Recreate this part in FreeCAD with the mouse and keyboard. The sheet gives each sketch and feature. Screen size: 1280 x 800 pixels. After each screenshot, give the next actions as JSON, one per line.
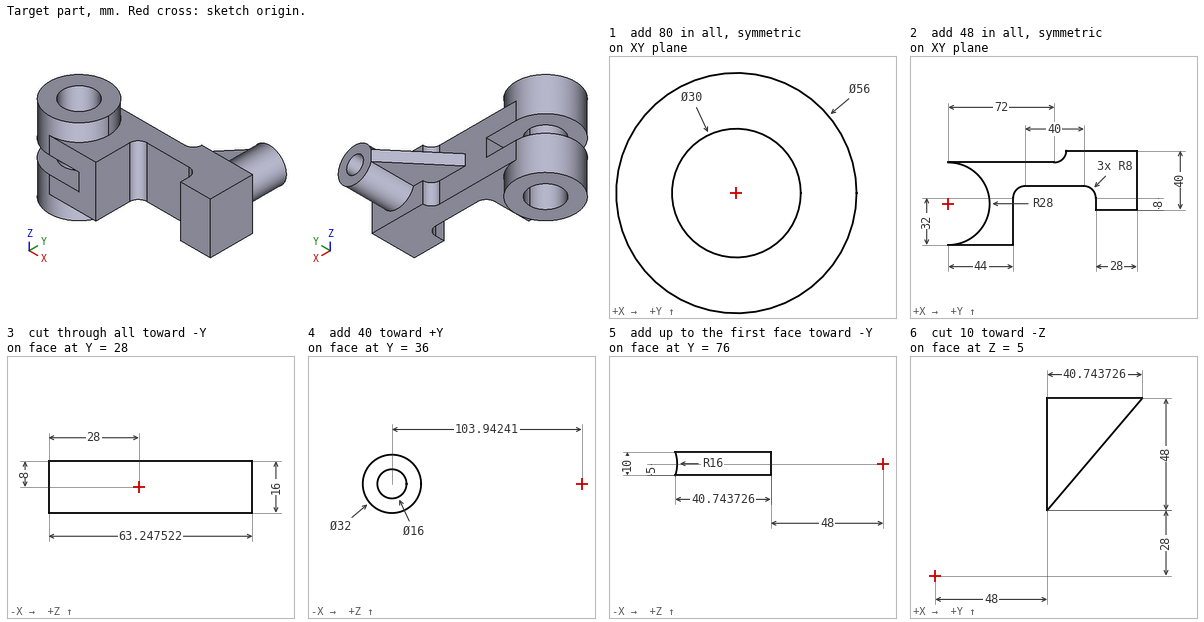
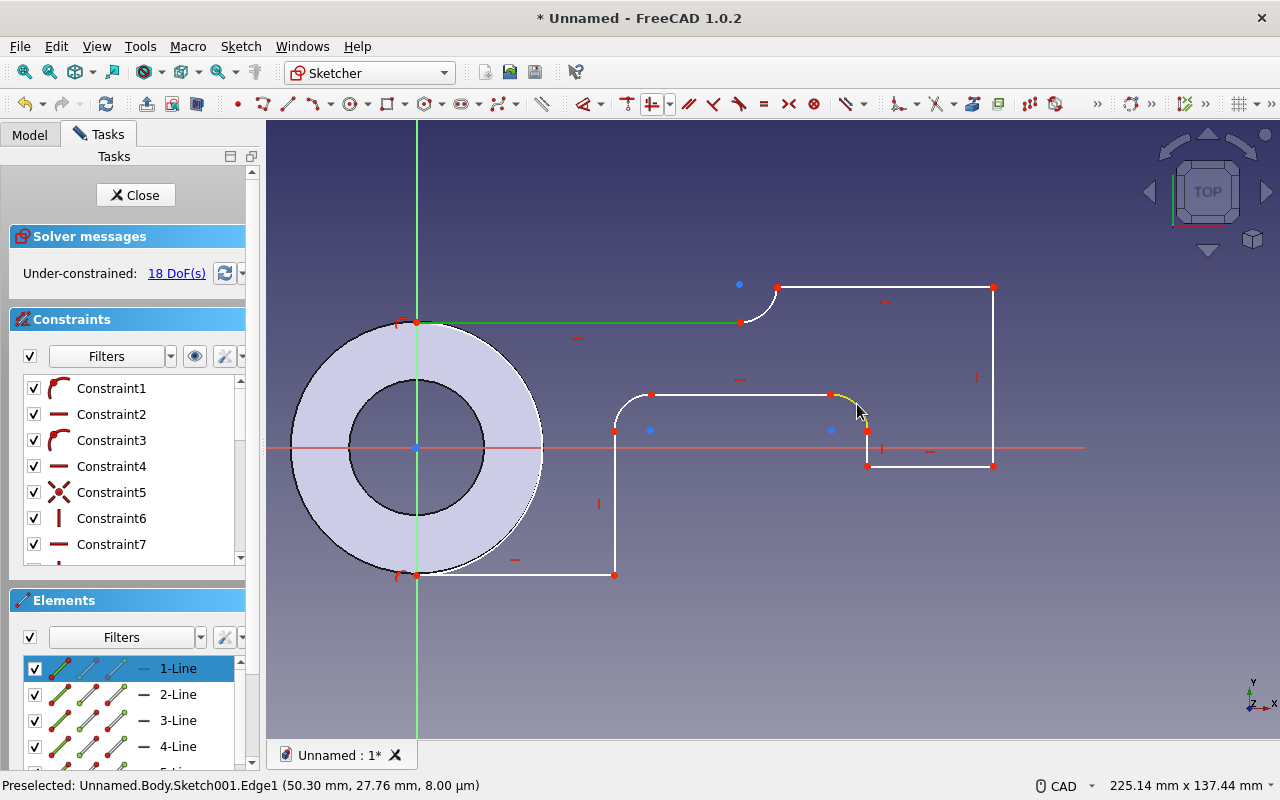
{"action": "left_click", "coordinate": [518, 523]}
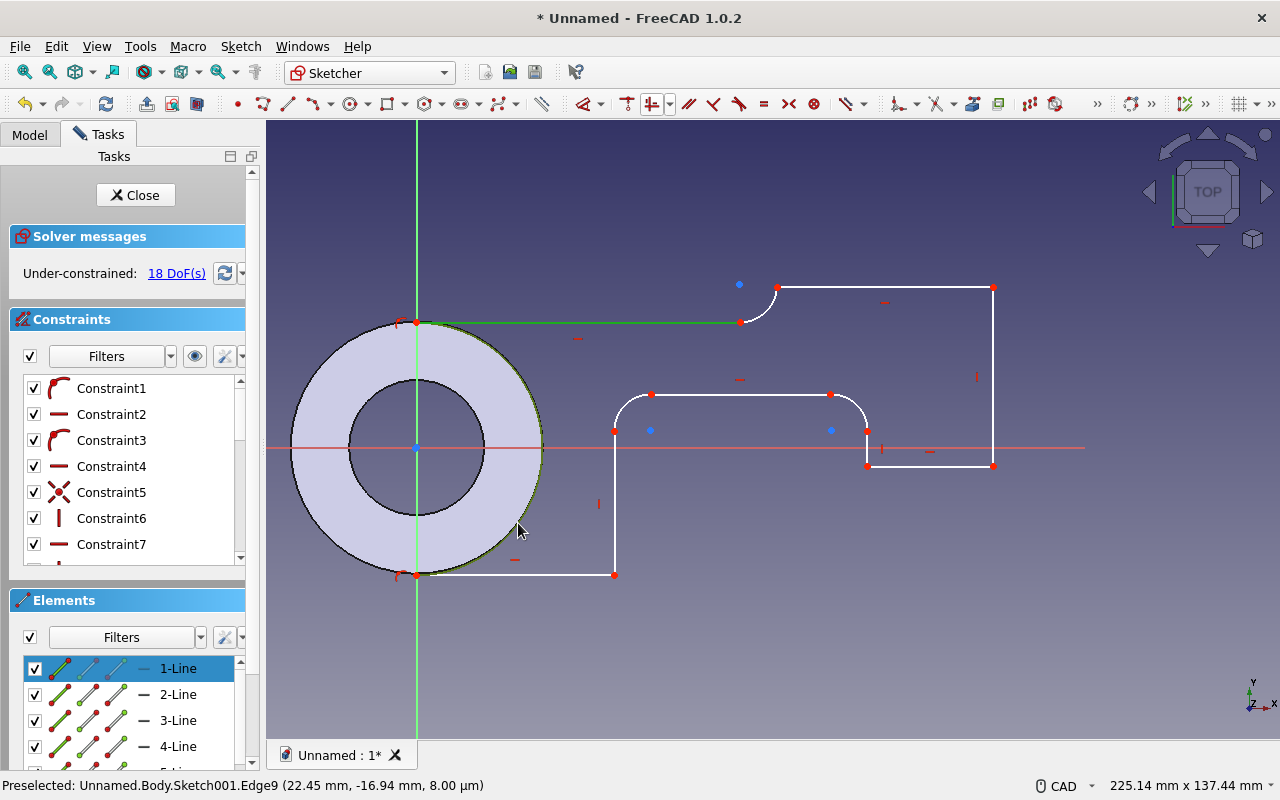
{"action": "left_click", "coordinate": [739, 104]}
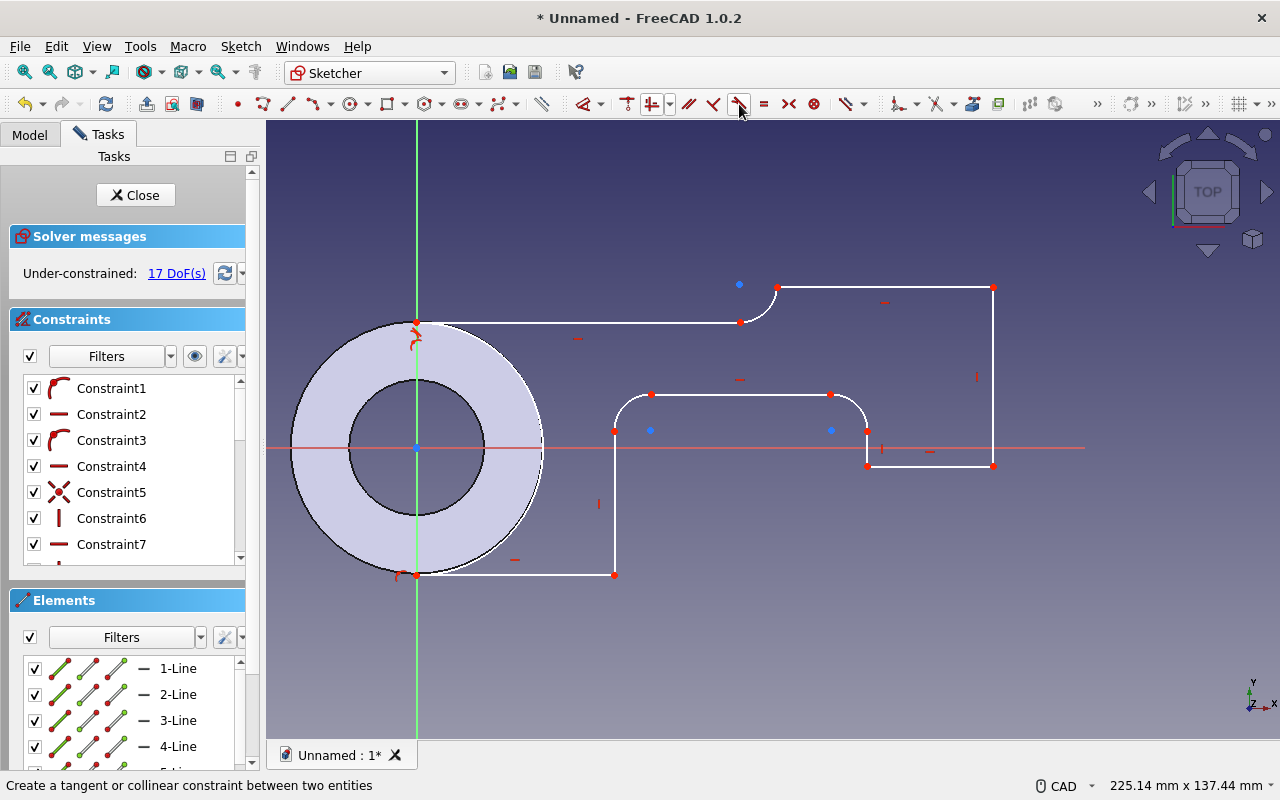
{"action": "left_click", "coordinate": [643, 323]}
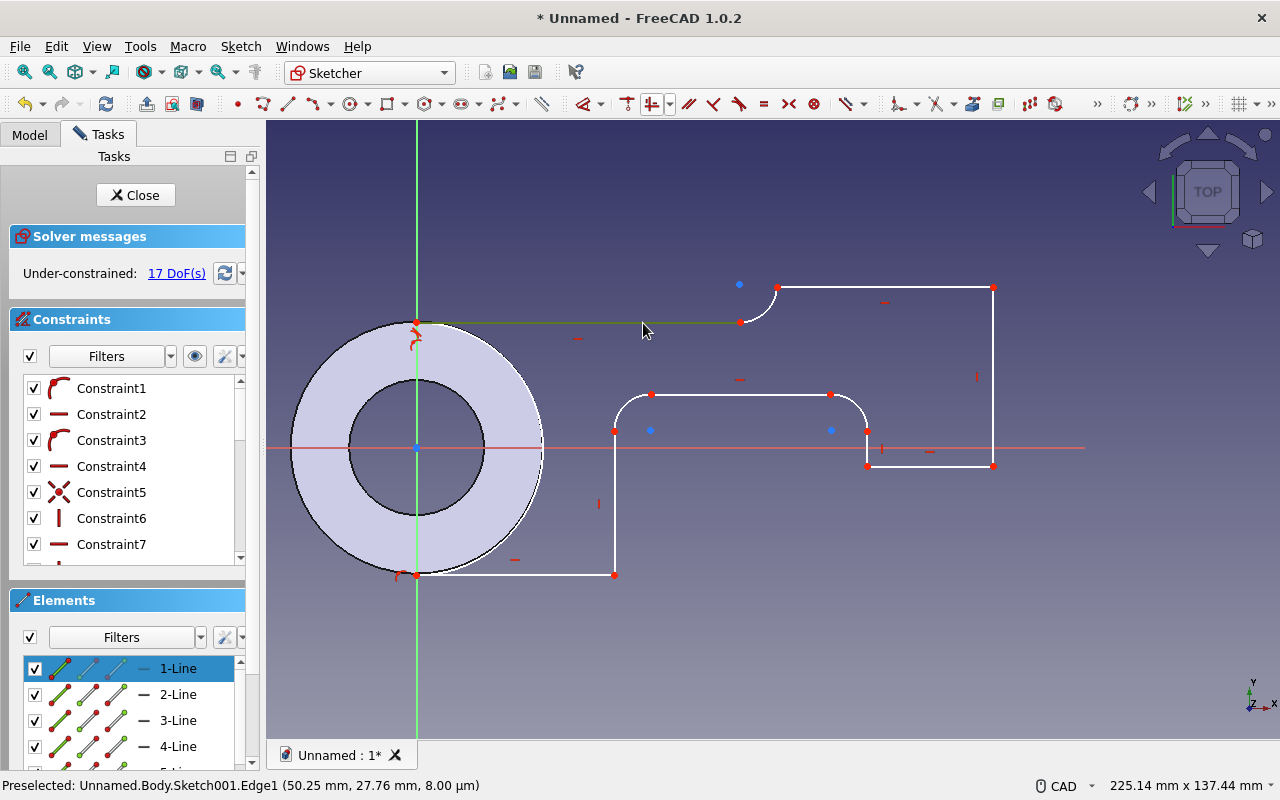
{"action": "left_click", "coordinate": [757, 318]}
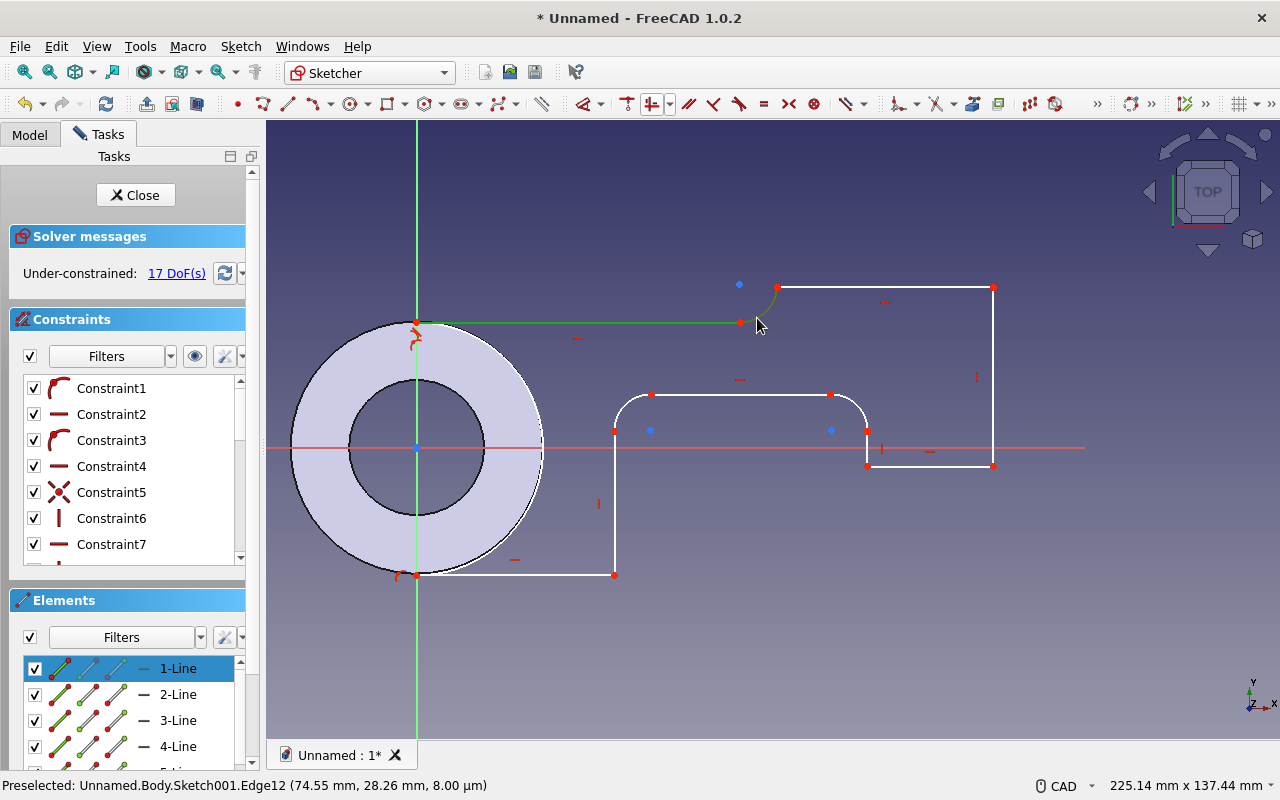
{"action": "left_click", "coordinate": [739, 104]}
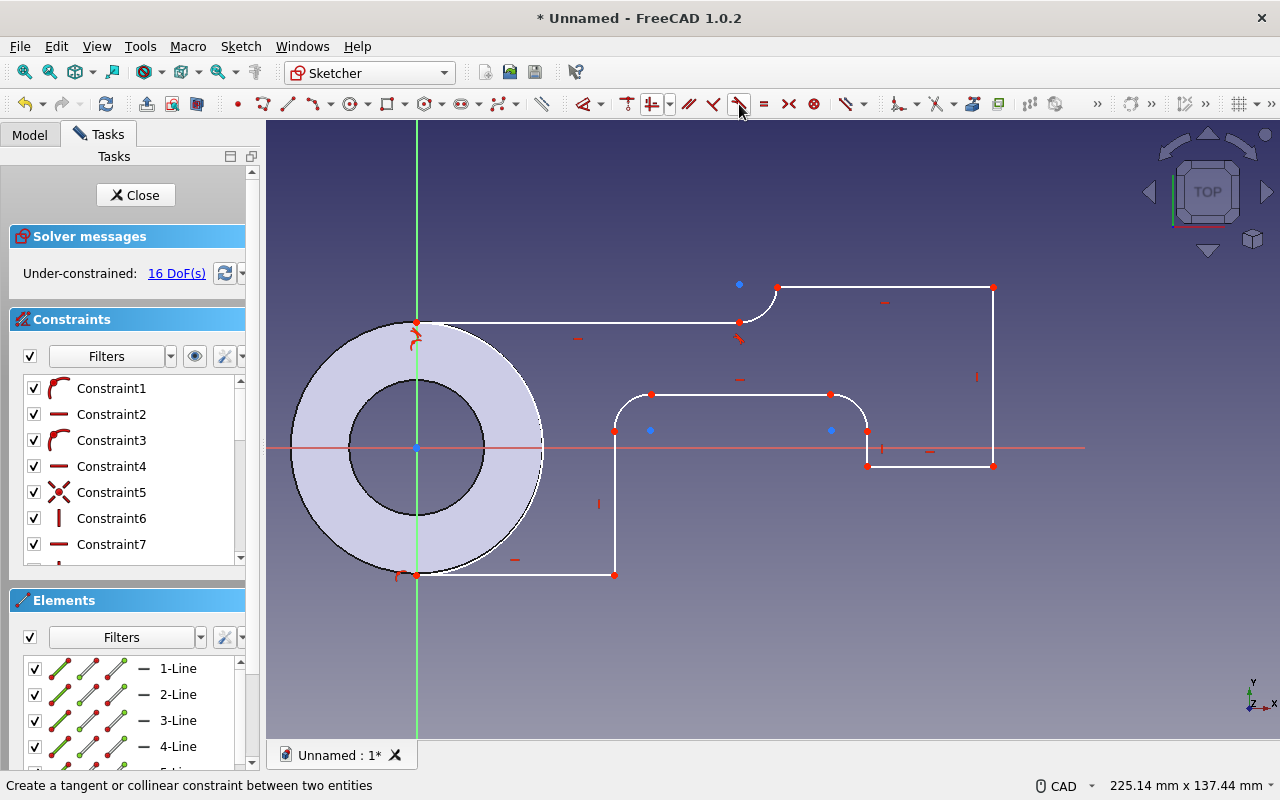
{"action": "left_click", "coordinate": [615, 532]}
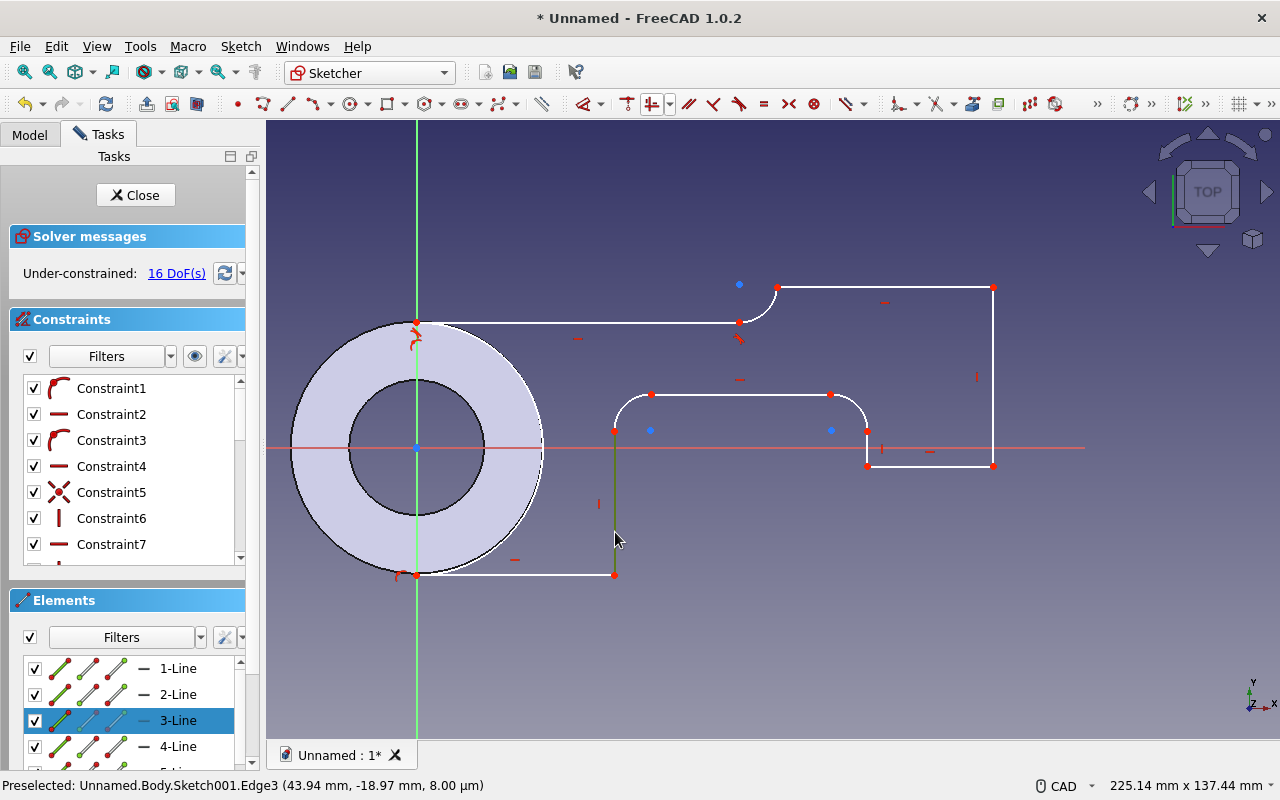
{"action": "left_click", "coordinate": [634, 398]}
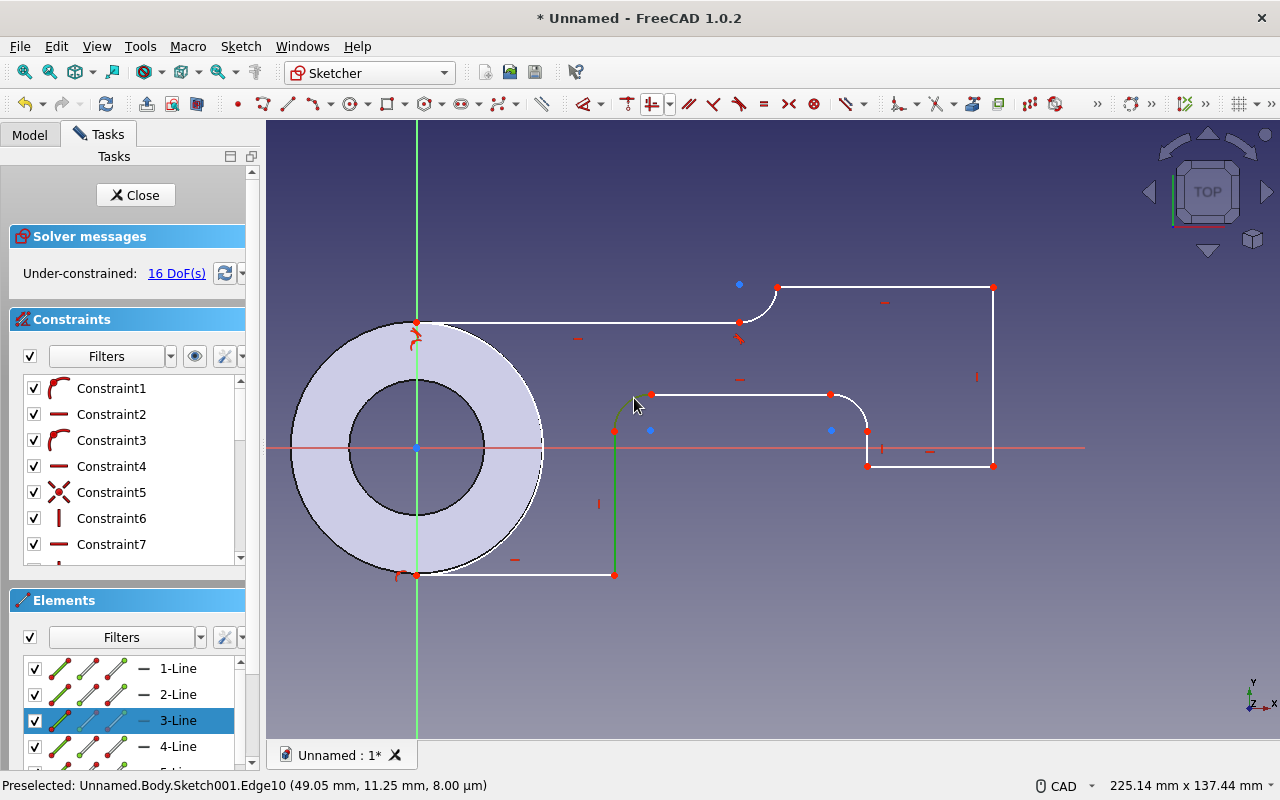
{"action": "key", "text": "t"}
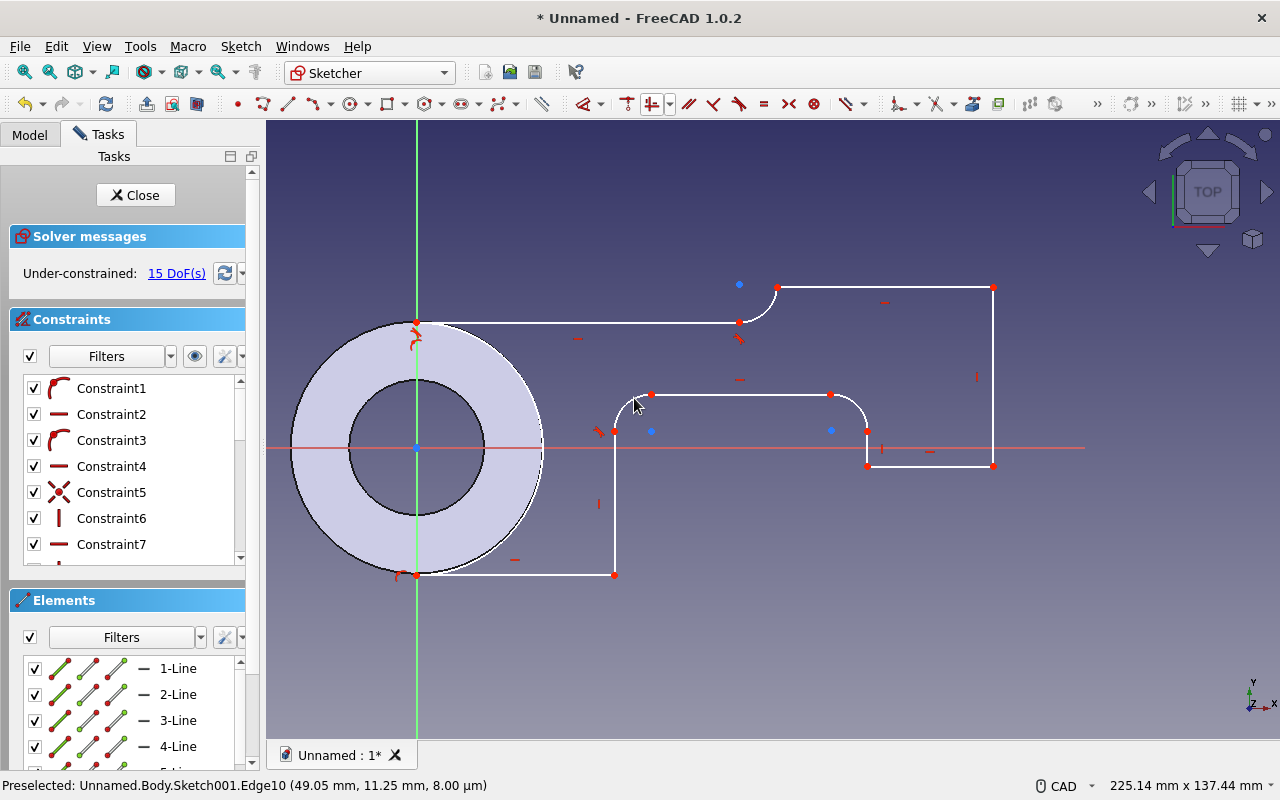
{"action": "left_click", "coordinate": [705, 395]}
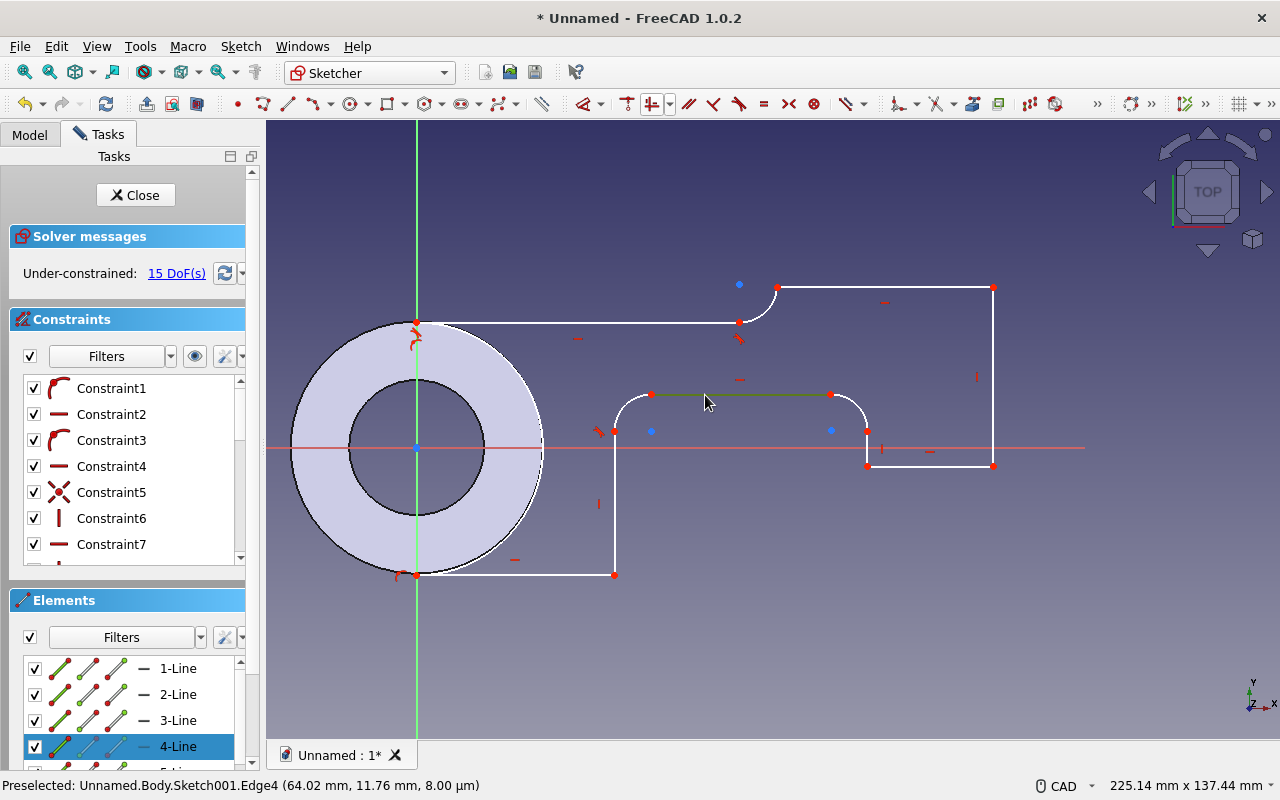
{"action": "left_click", "coordinate": [635, 399]}